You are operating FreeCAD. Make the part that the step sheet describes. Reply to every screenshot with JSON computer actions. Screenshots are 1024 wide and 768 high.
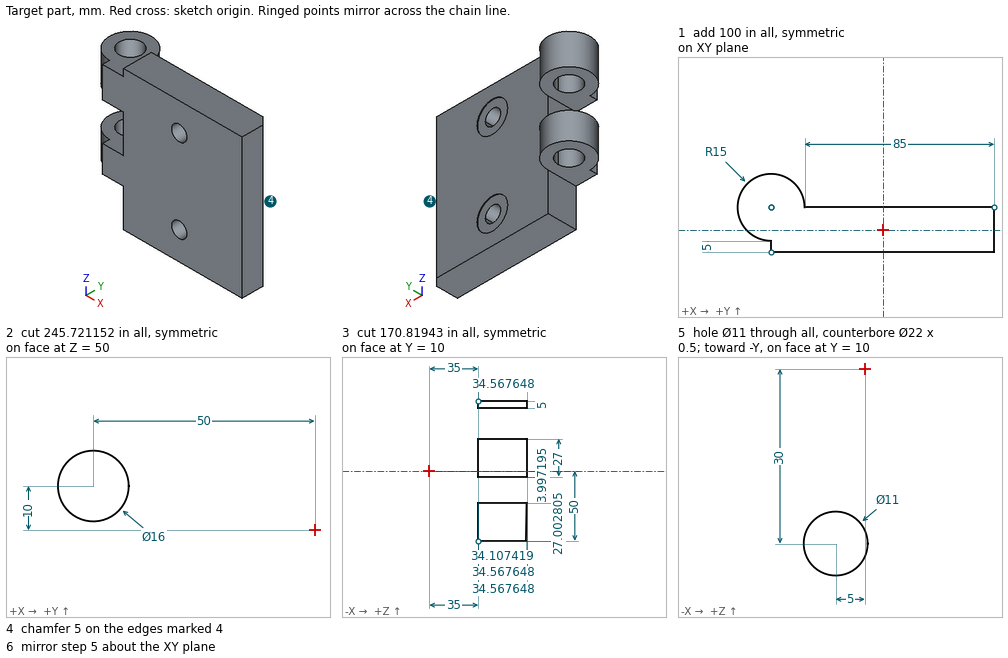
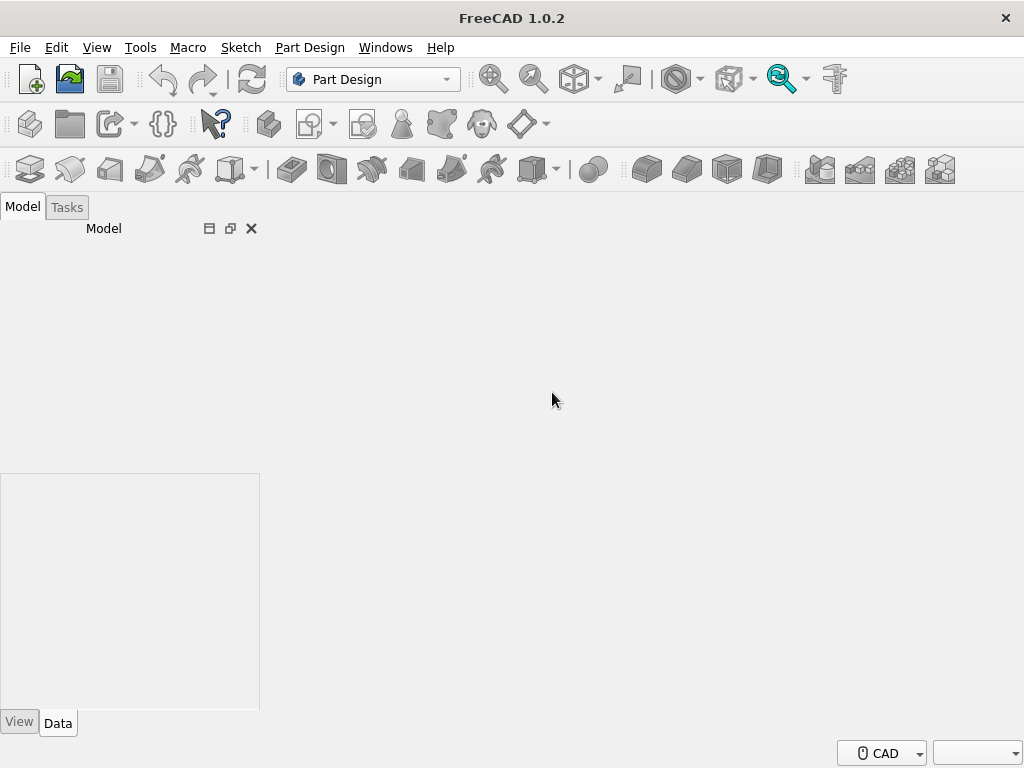
{"action": "left_click", "coordinate": [30, 80]}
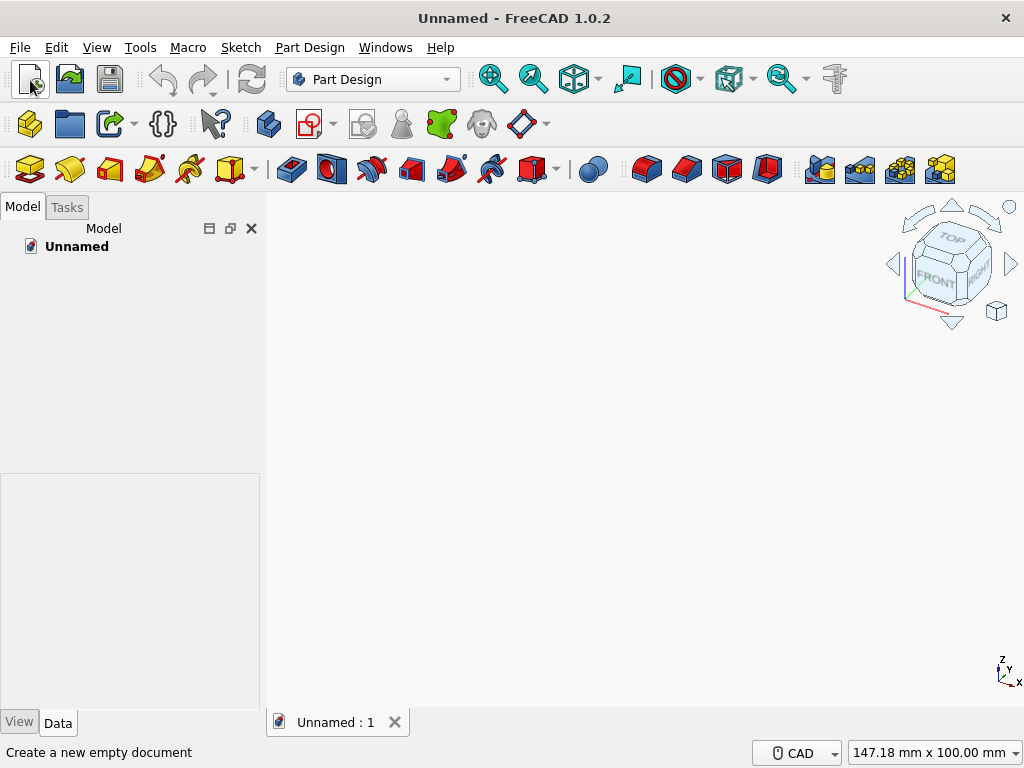
{"action": "left_click", "coordinate": [310, 124]}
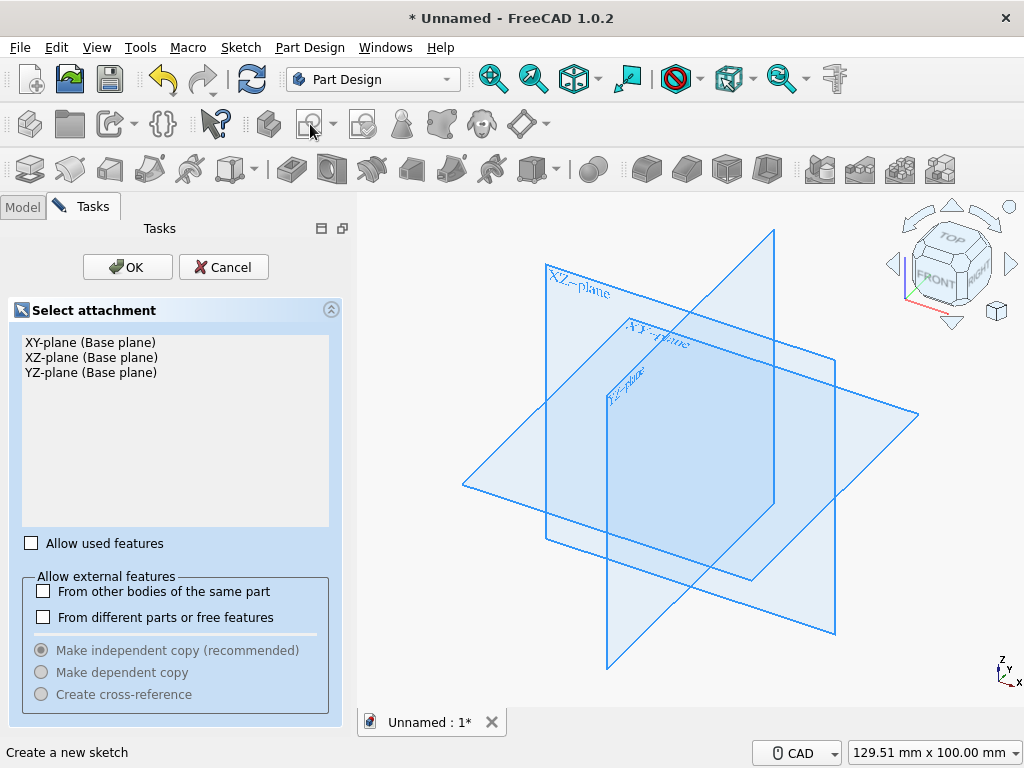
{"action": "left_click", "coordinate": [82, 342]}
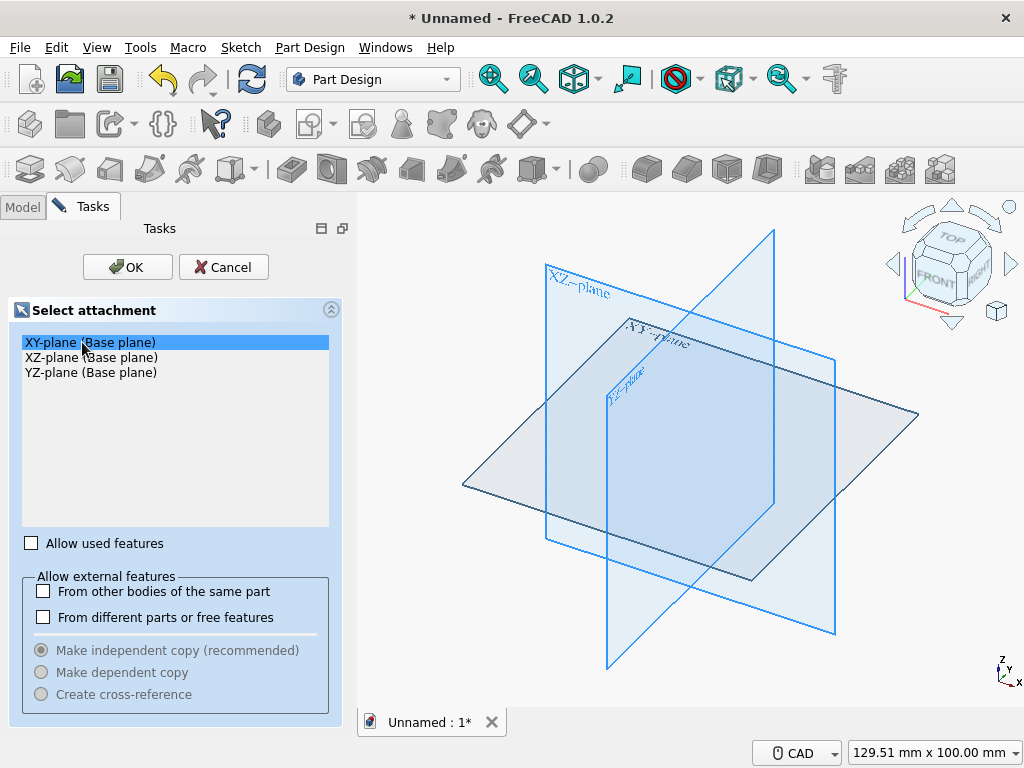
{"action": "left_click", "coordinate": [128, 267]}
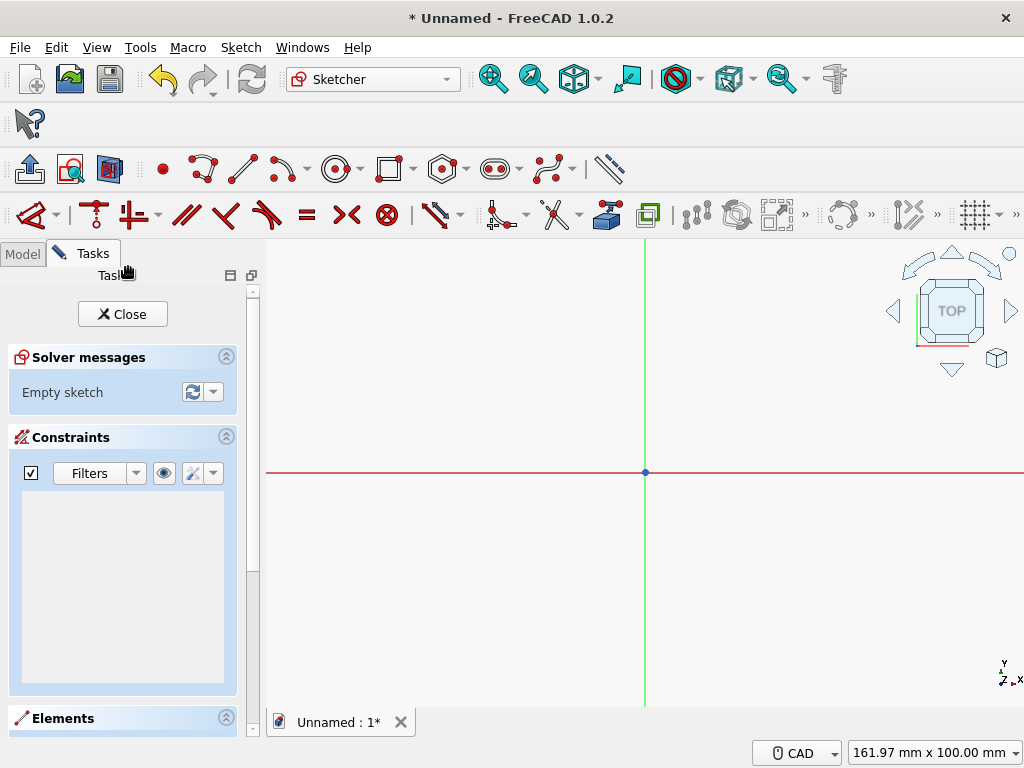
{"action": "scroll", "coordinate": [379, 585], "scroll_direction": "down", "scroll_amount": 1}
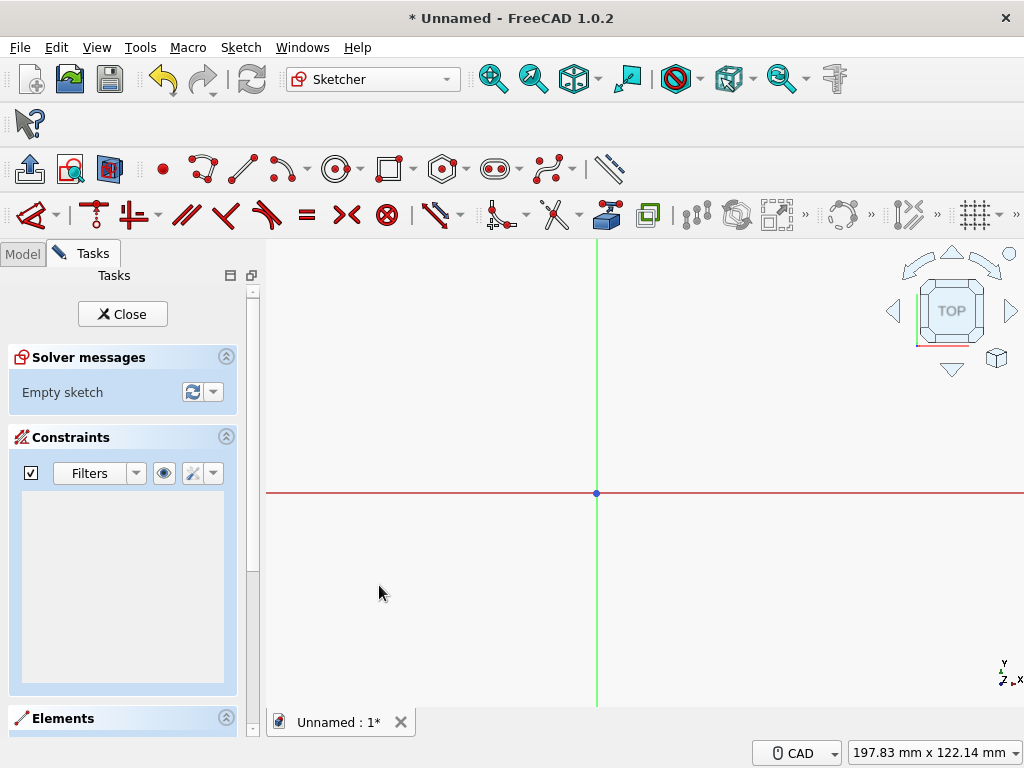
{"action": "left_click", "coordinate": [204, 170]}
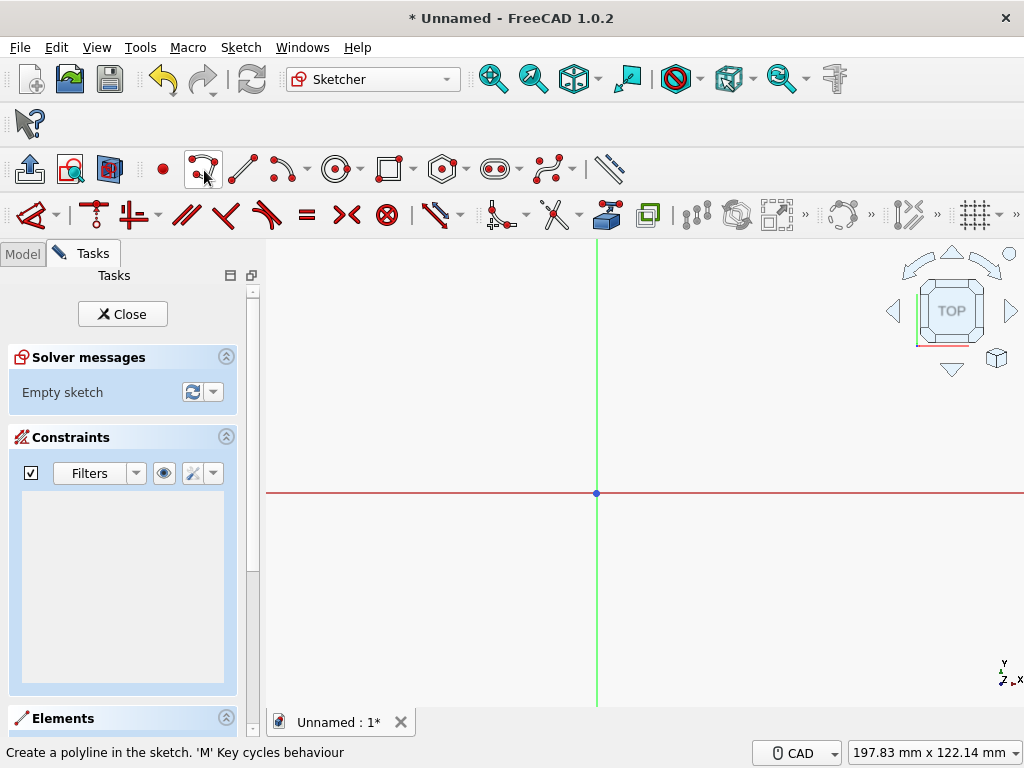
{"action": "left_click", "coordinate": [405, 513]}
{"action": "left_click", "coordinate": [405, 532]}
{"action": "left_click", "coordinate": [788, 532]}
{"action": "left_click", "coordinate": [788, 455]}
{"action": "left_click", "coordinate": [463, 455]}
{"action": "right_click", "coordinate": [463, 455]}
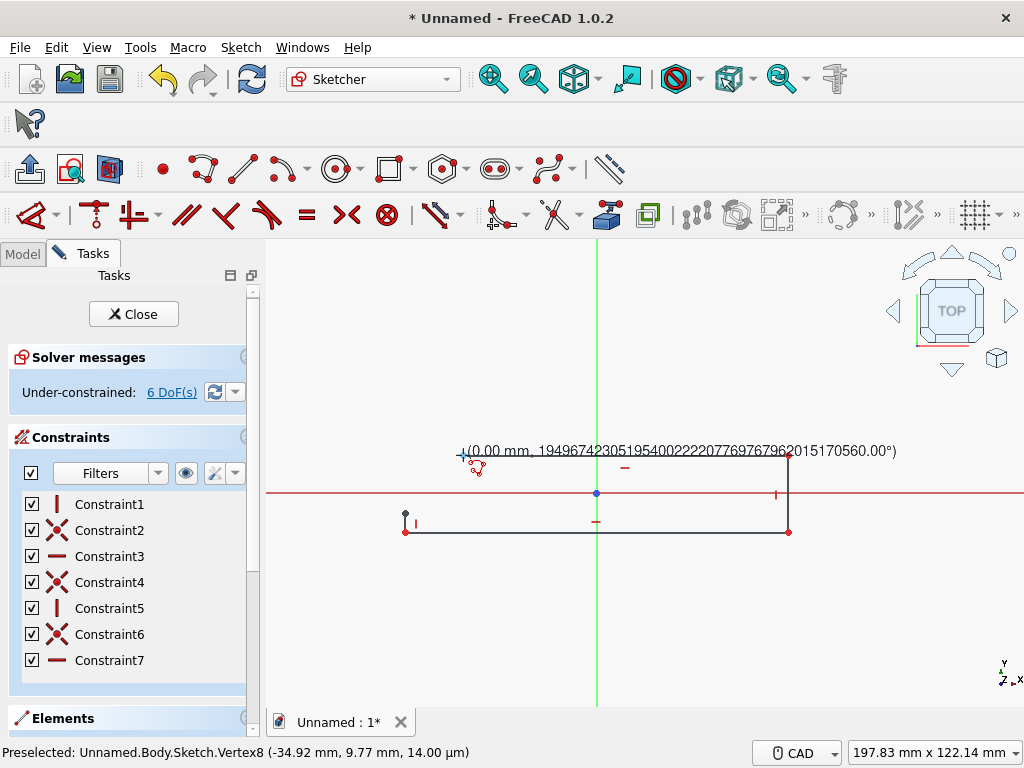
{"action": "left_click", "coordinate": [310, 170]}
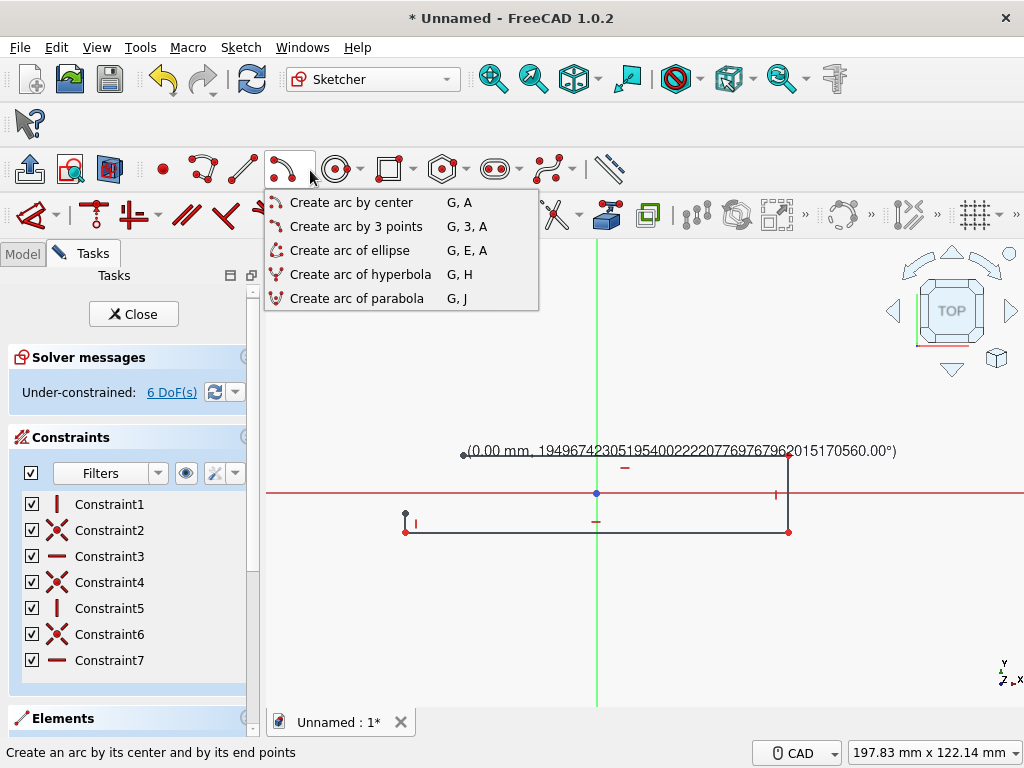
{"action": "left_click", "coordinate": [402, 226]}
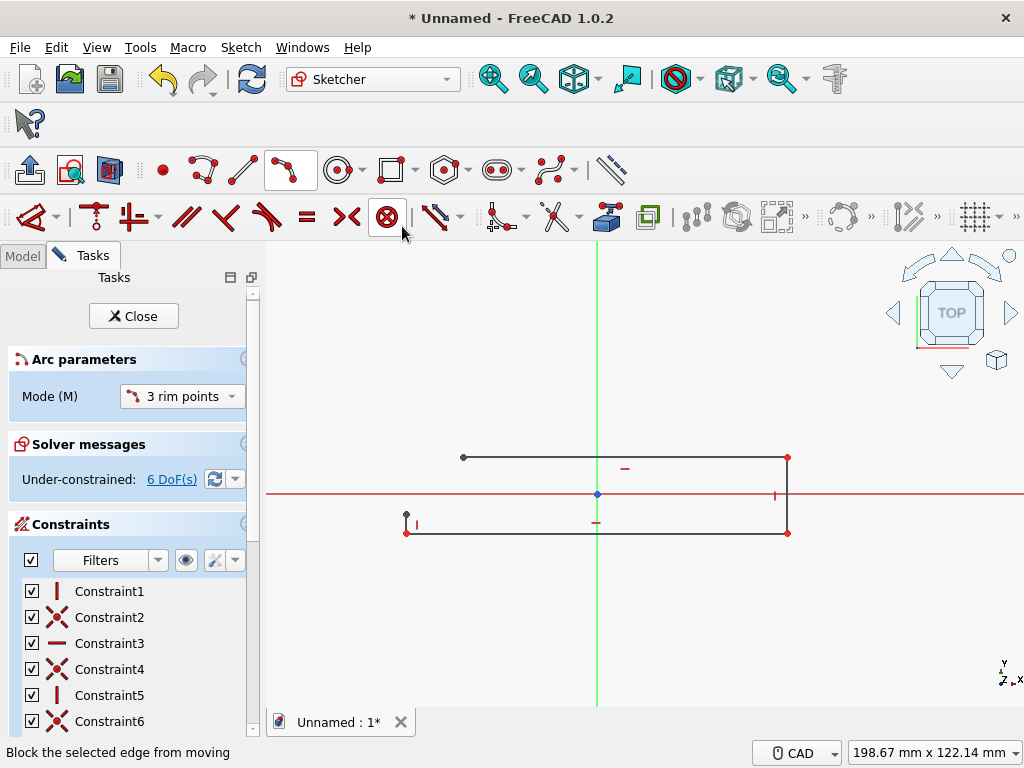
{"action": "left_click", "coordinate": [464, 457]}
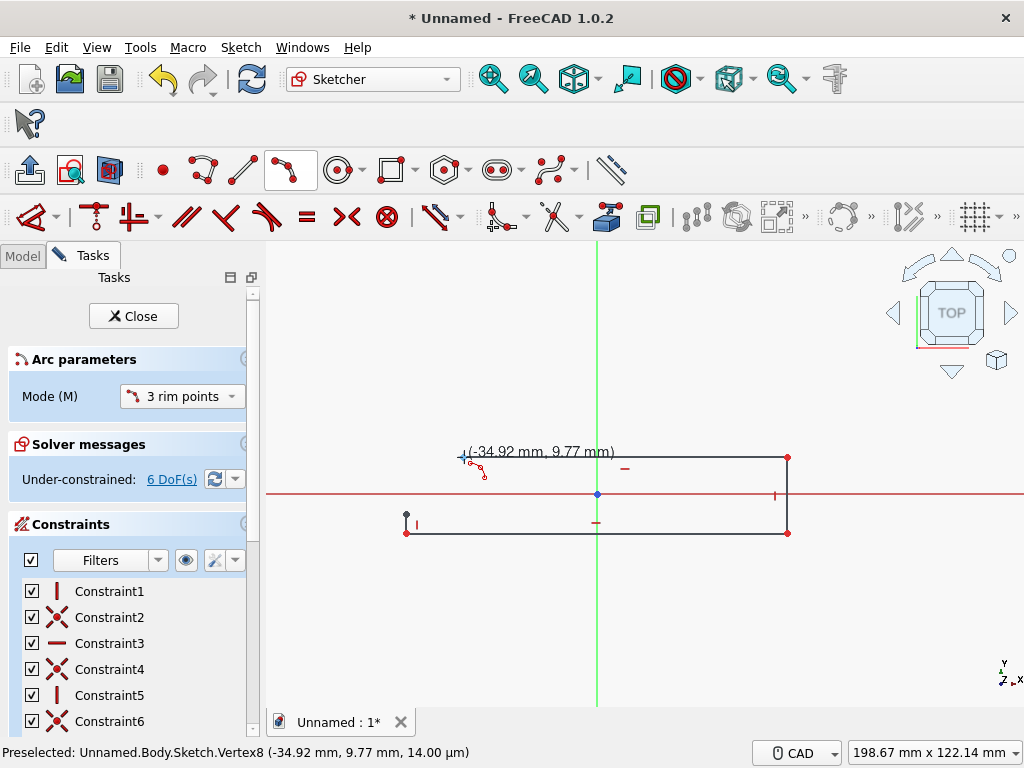
{"action": "scroll", "coordinate": [406, 513], "scroll_direction": "up", "scroll_amount": 3}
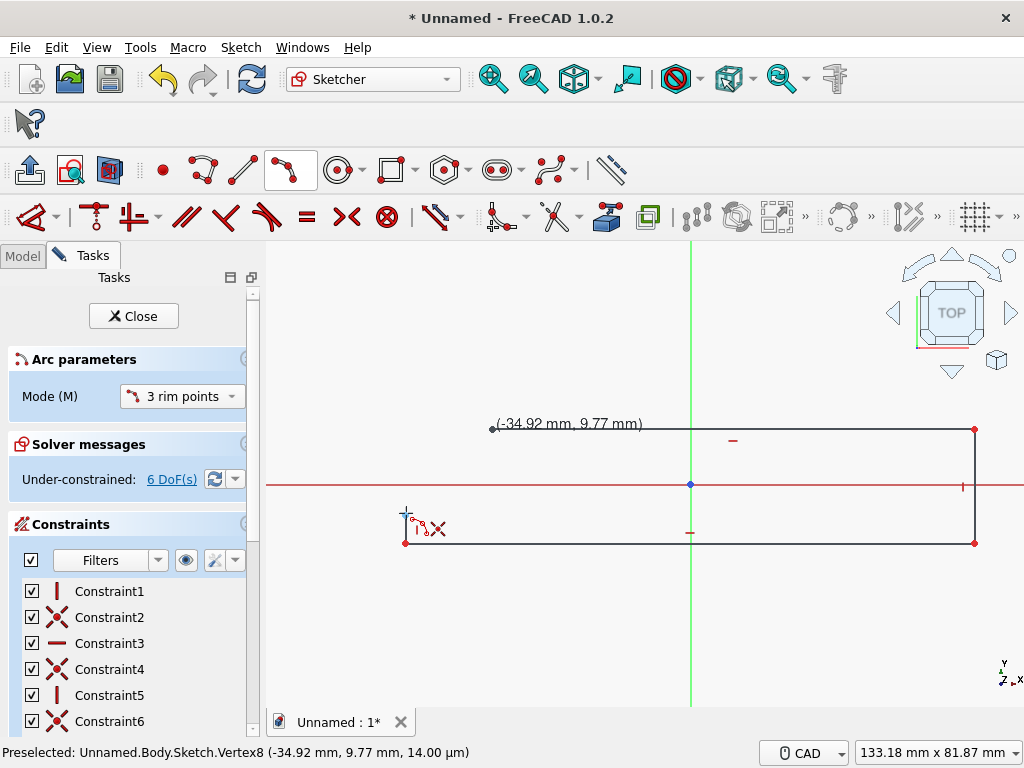
{"action": "left_click", "coordinate": [406, 516]}
{"action": "left_click", "coordinate": [333, 335]}
{"action": "key", "text": "Escape"}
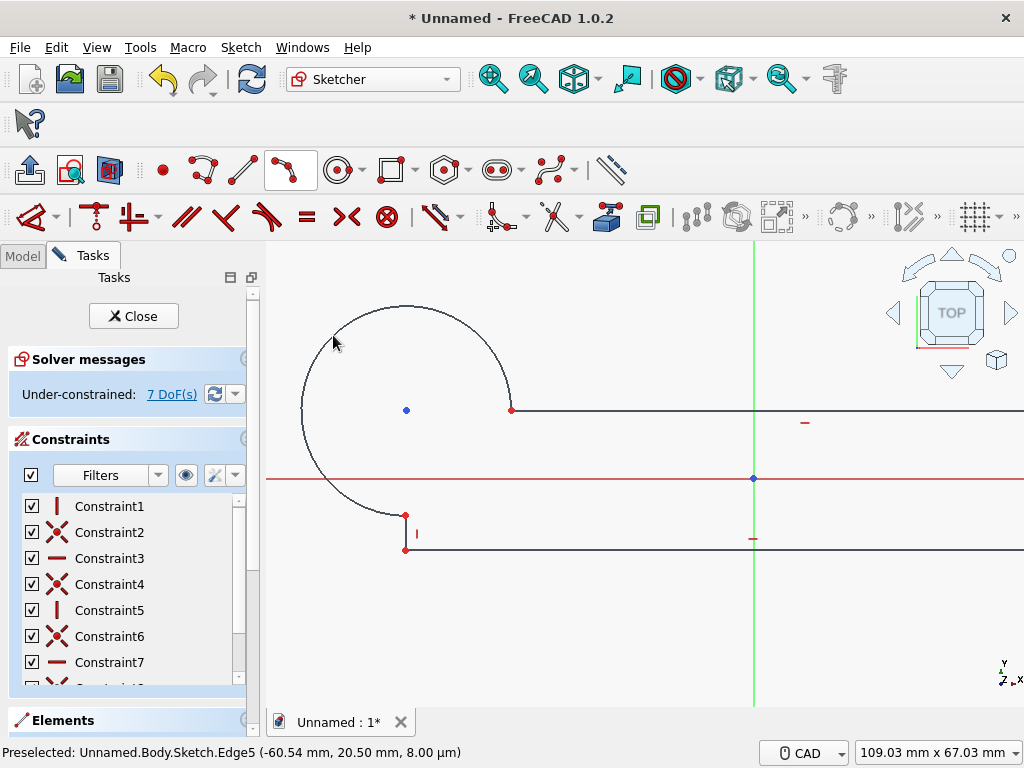
{"action": "left_click", "coordinate": [406, 411]}